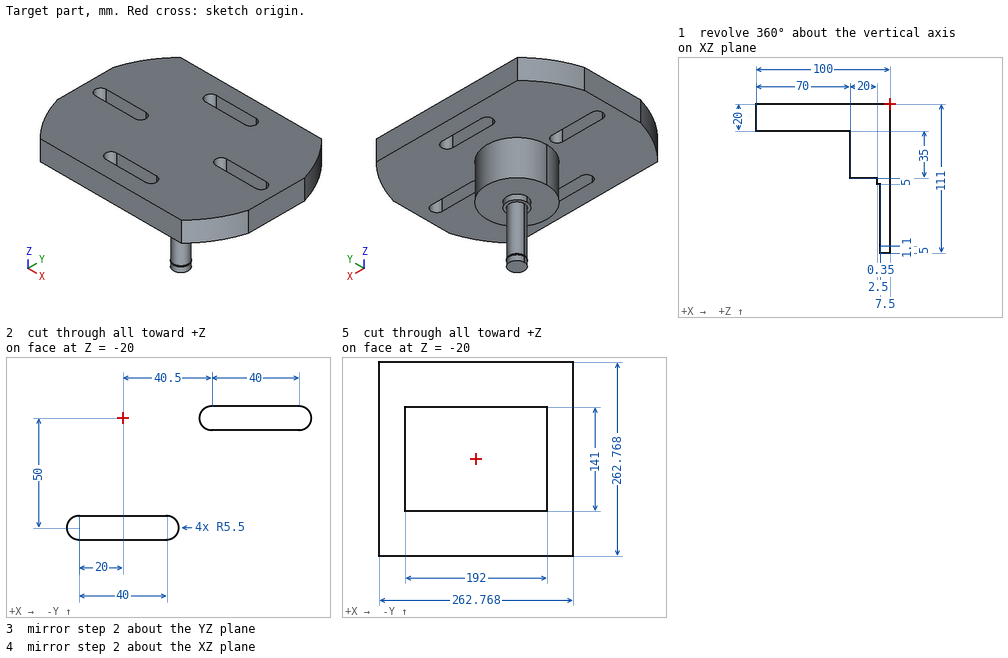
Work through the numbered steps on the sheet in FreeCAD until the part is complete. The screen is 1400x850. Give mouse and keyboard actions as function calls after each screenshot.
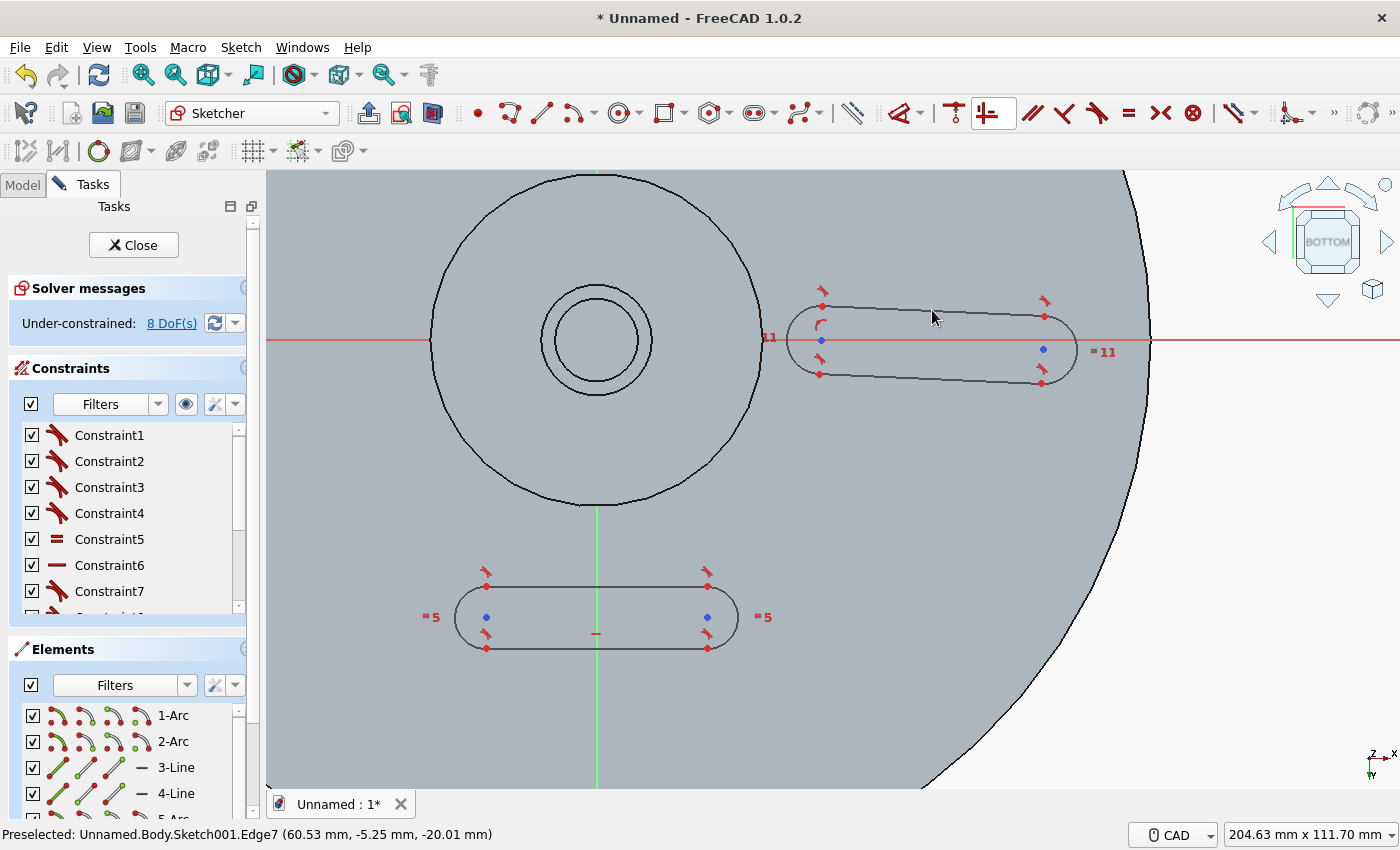
click(889, 309)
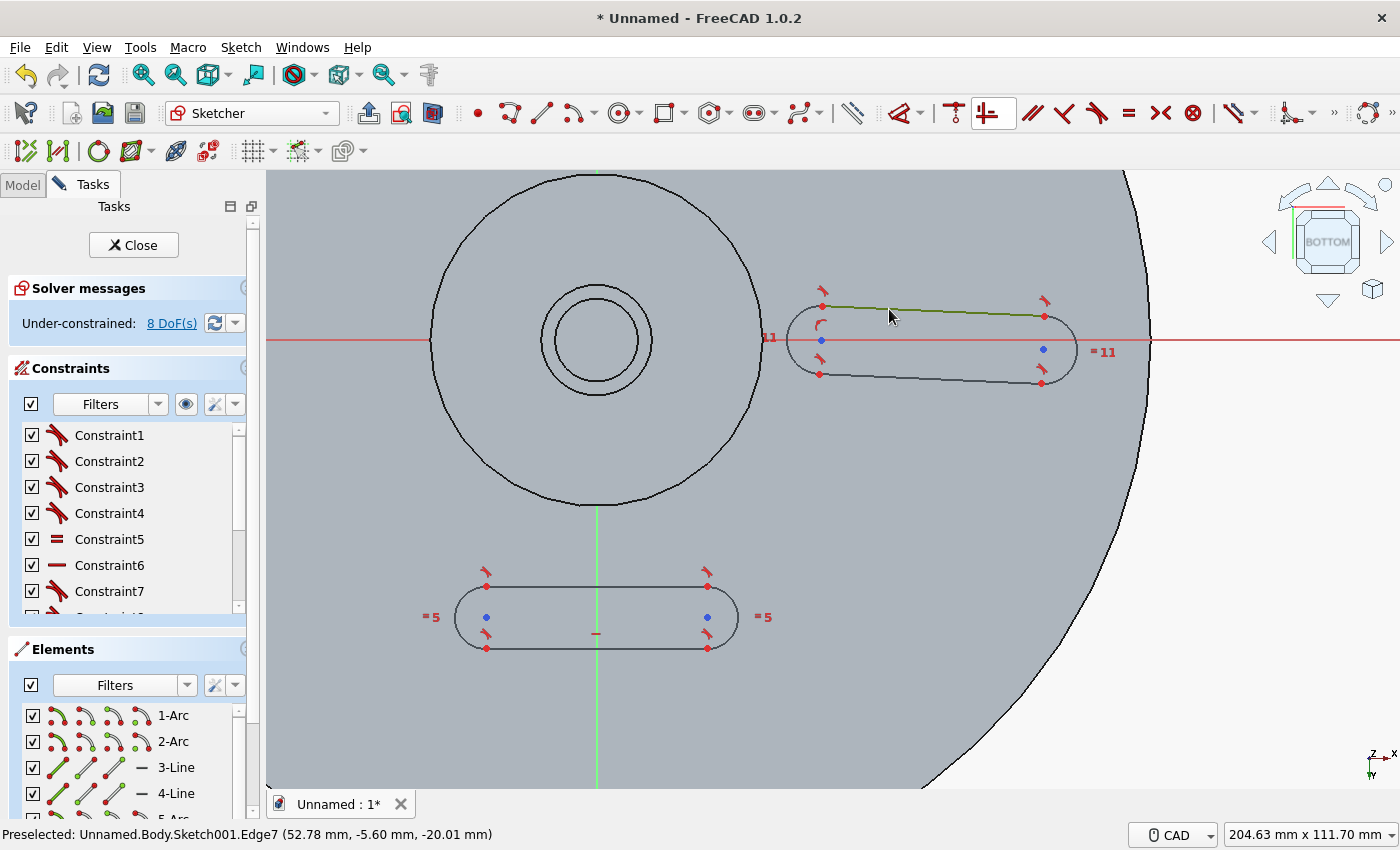
click(1010, 114)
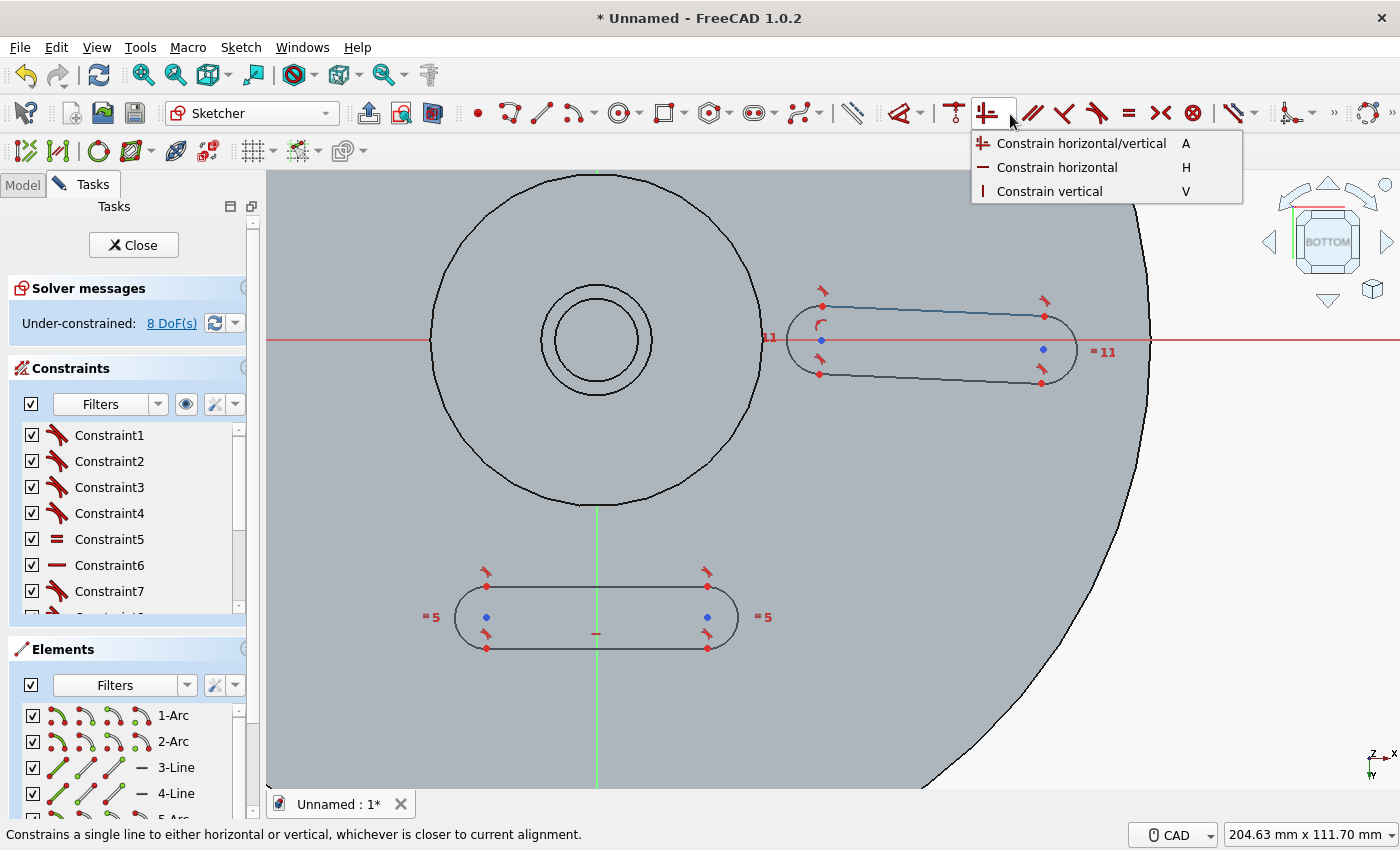
click(1107, 167)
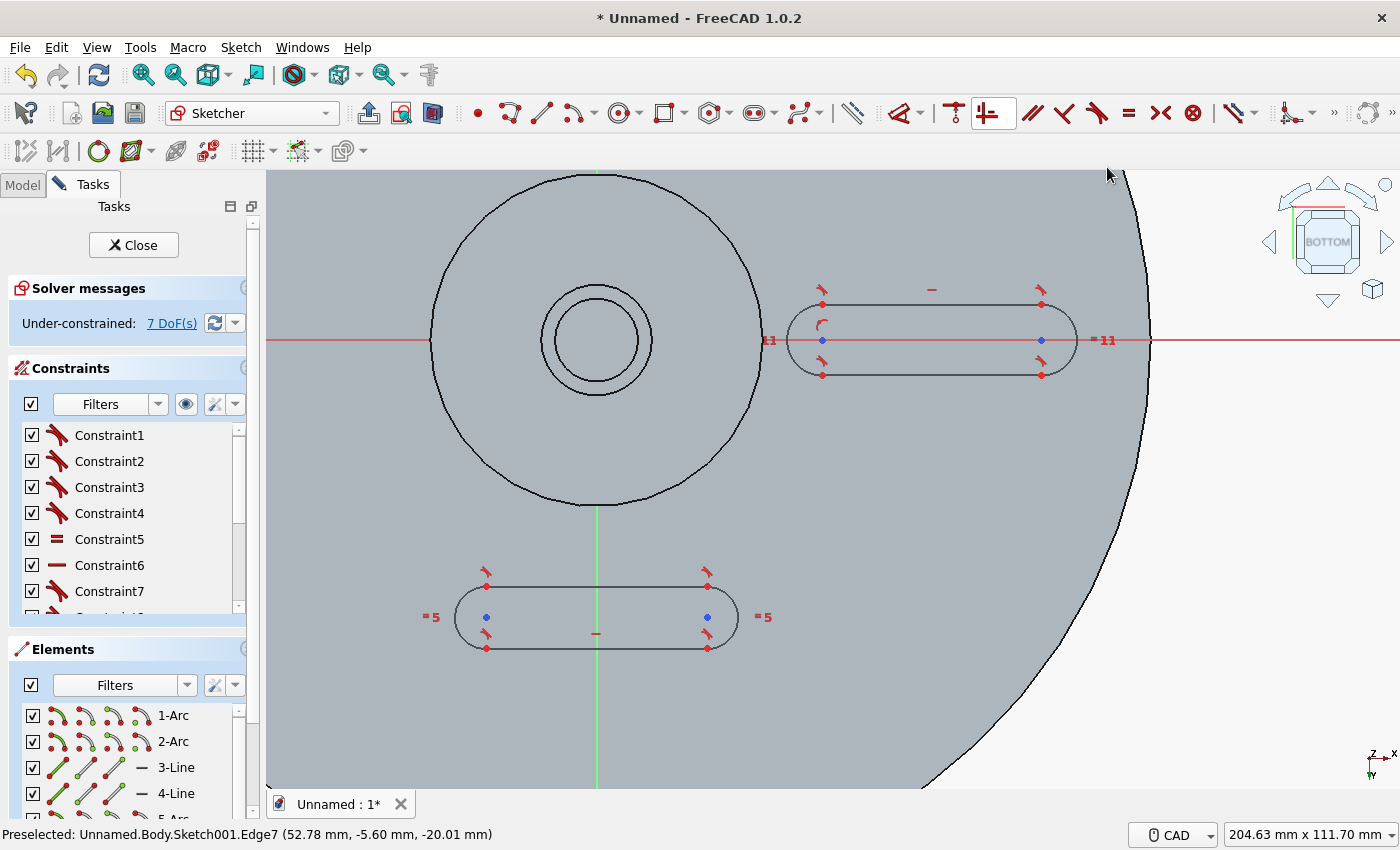
click(461, 600)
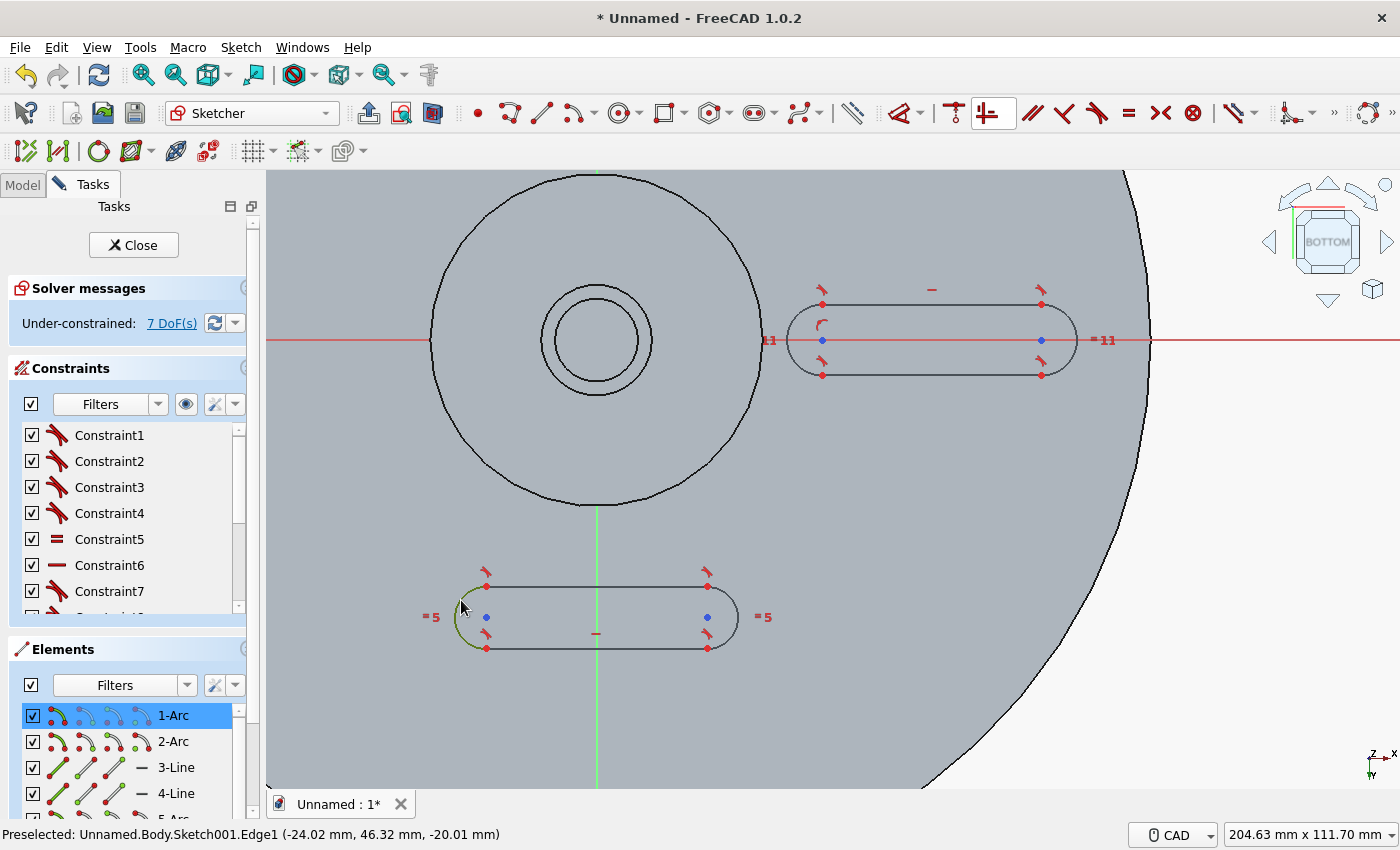
click(794, 319)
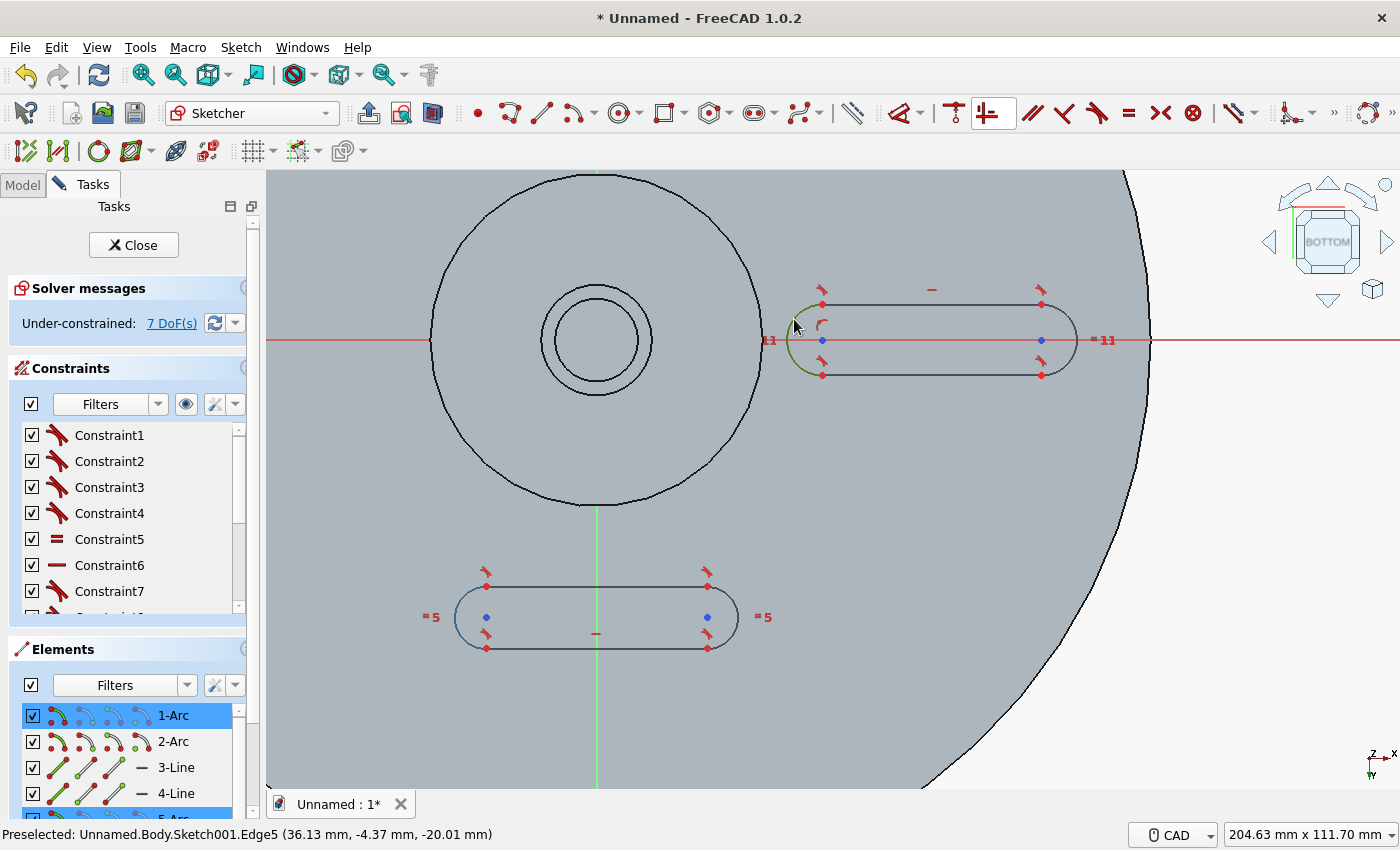
click(1130, 114)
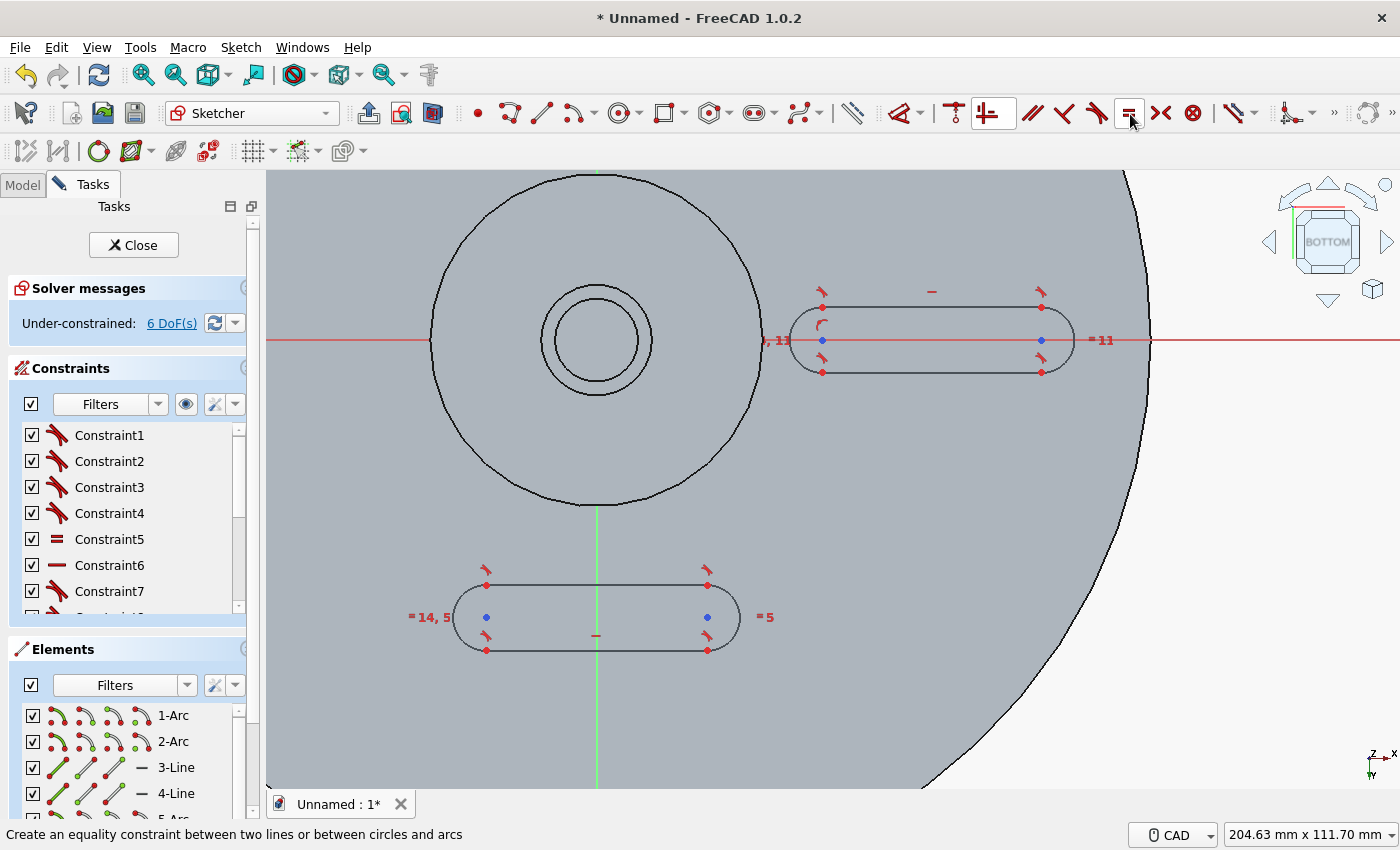
click(900, 114)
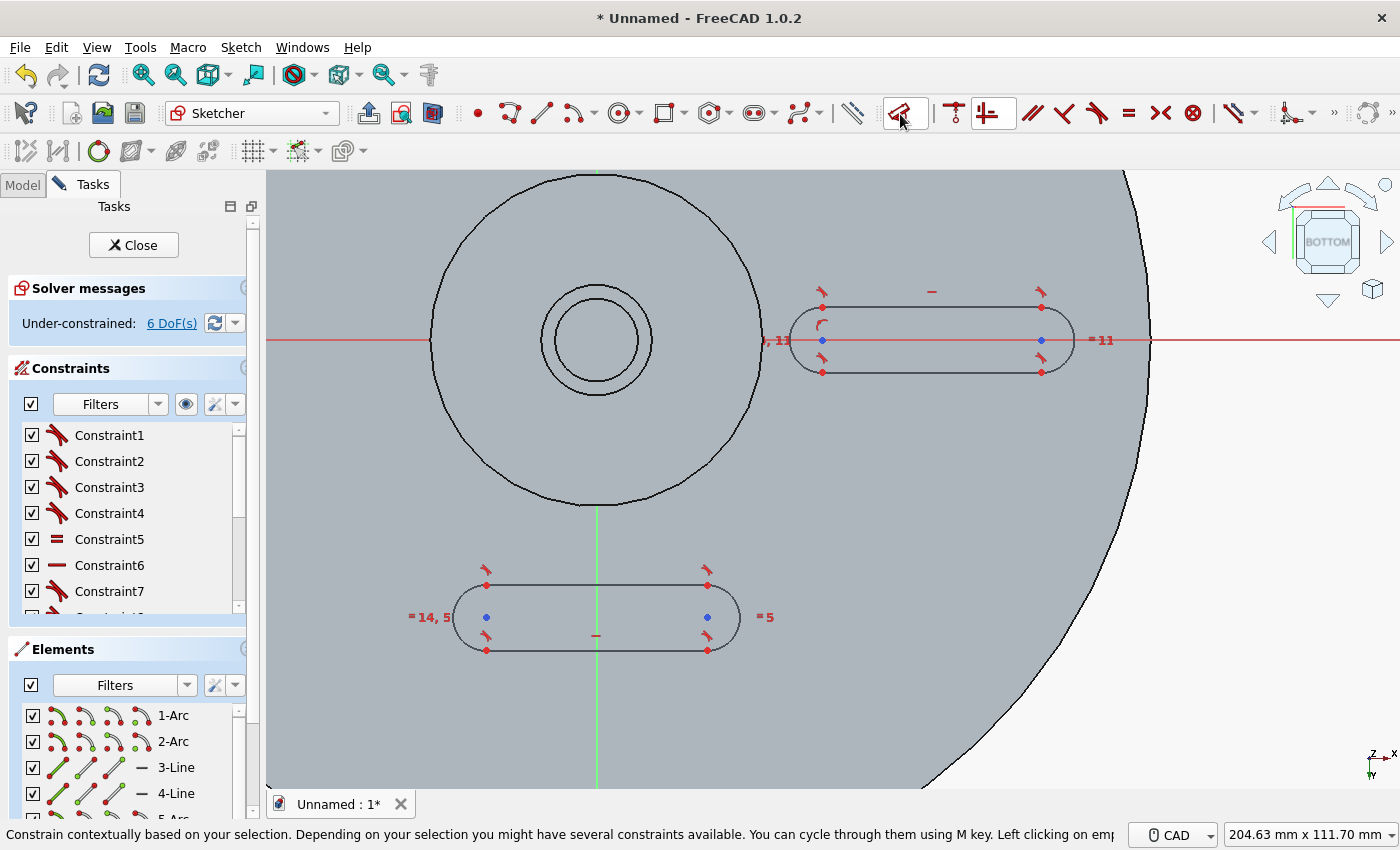
scroll(459, 599, up, 2)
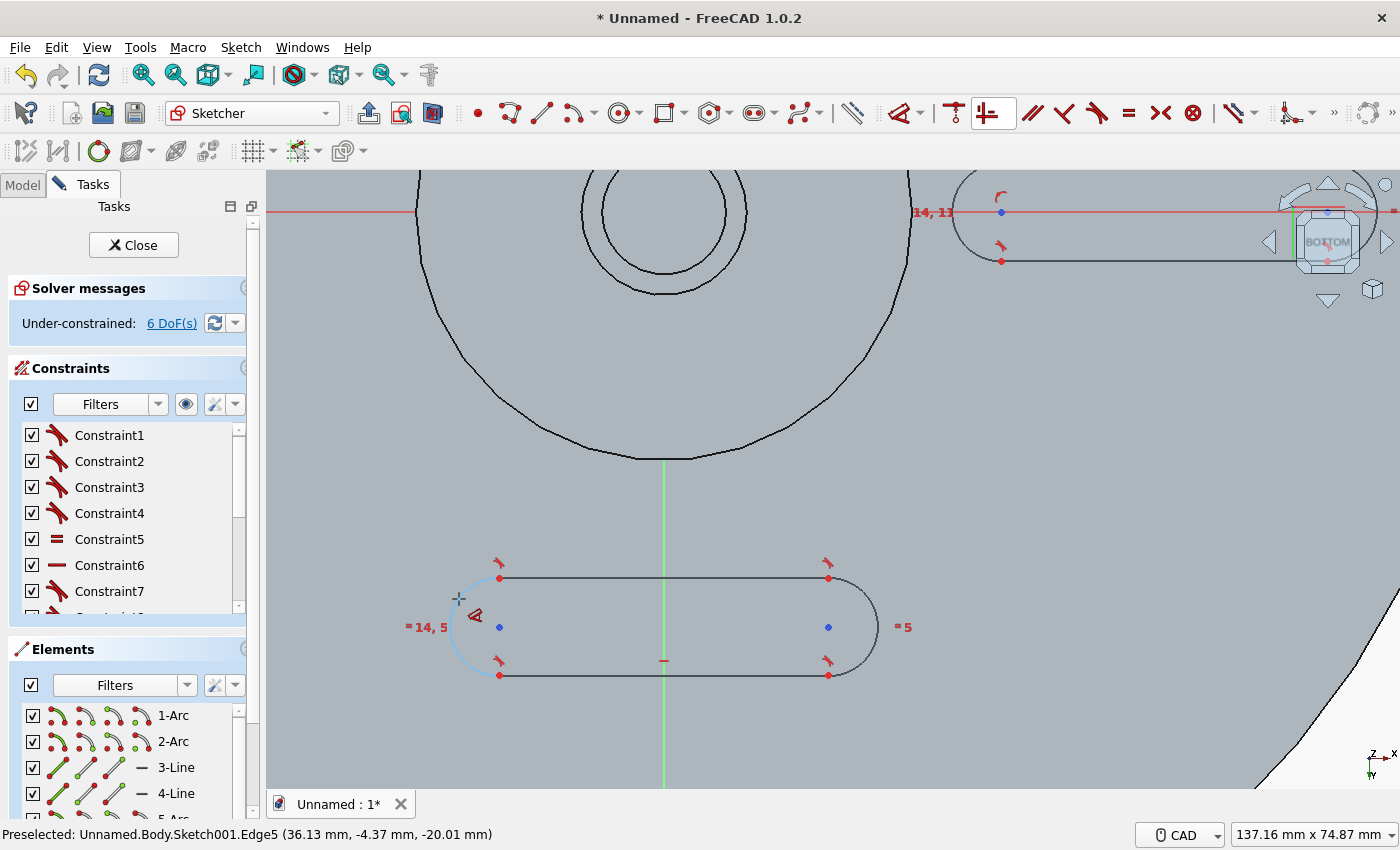
click(460, 598)
click(434, 579)